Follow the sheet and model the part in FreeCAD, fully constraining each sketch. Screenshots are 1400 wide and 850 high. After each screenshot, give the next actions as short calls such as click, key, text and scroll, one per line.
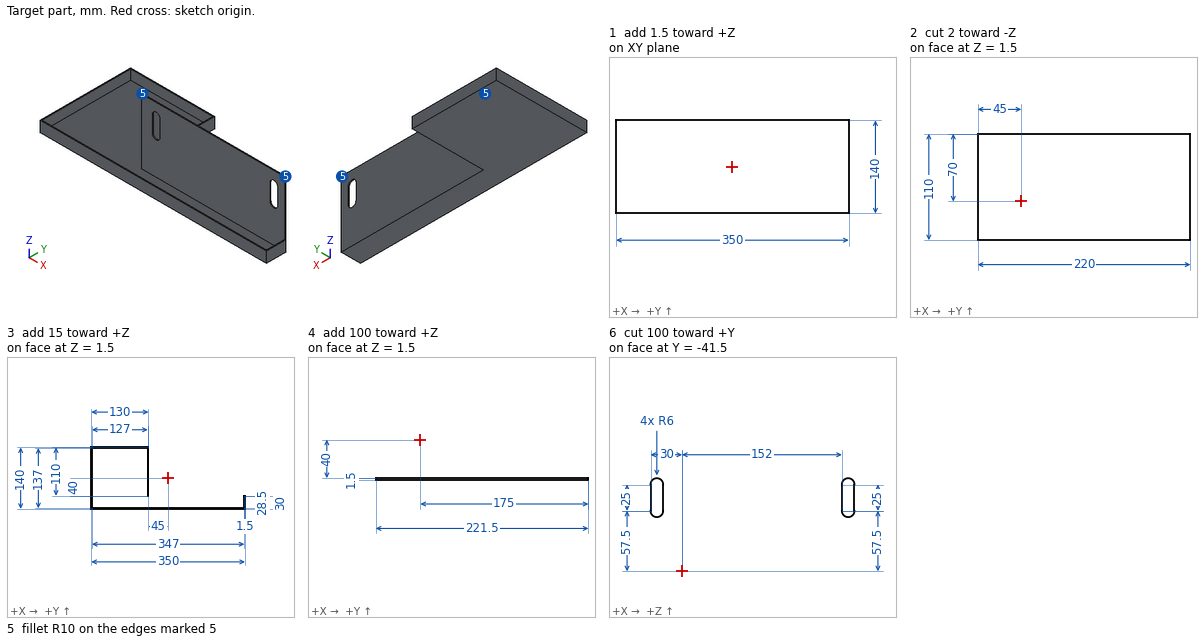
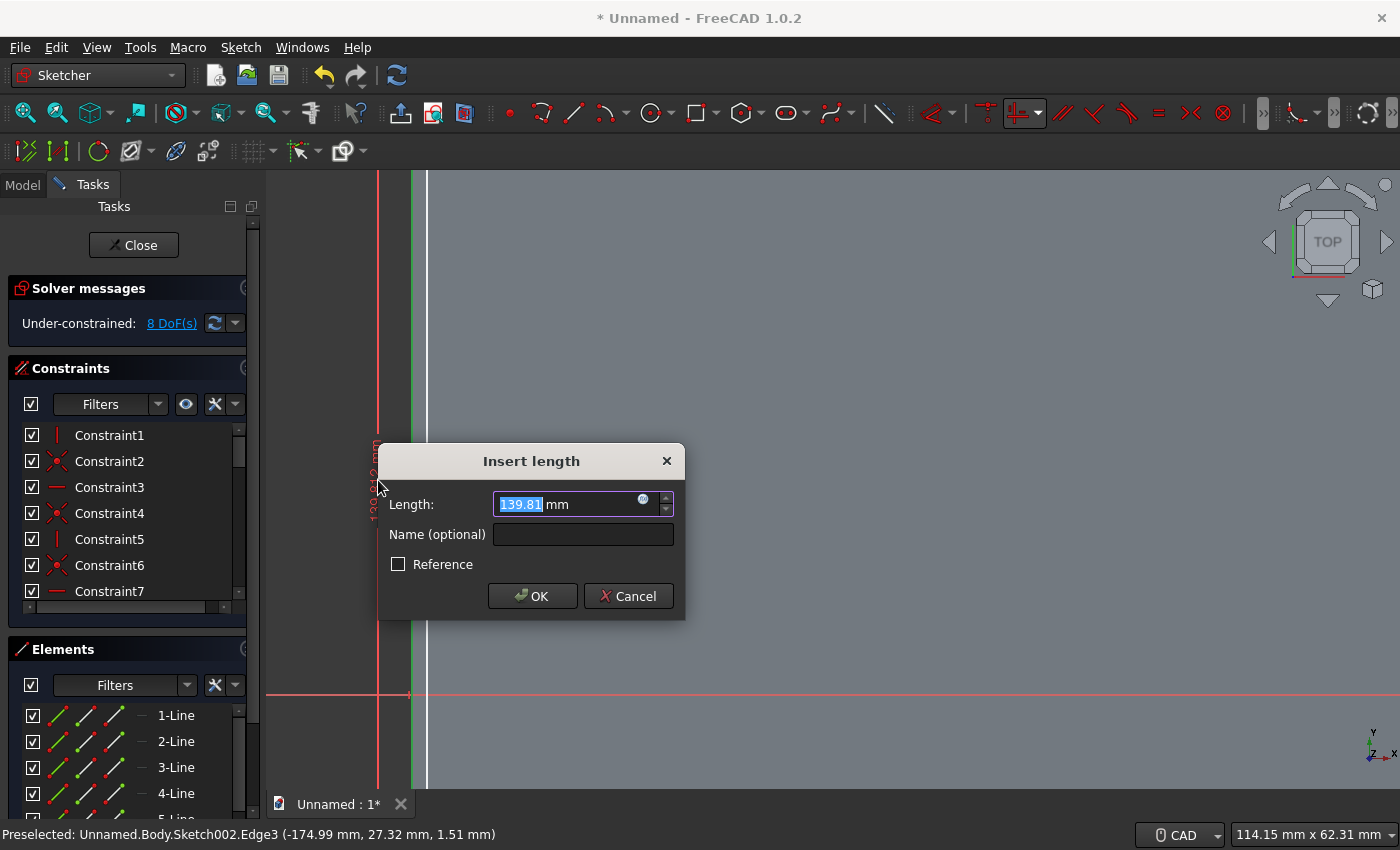
text(140)
key(Return)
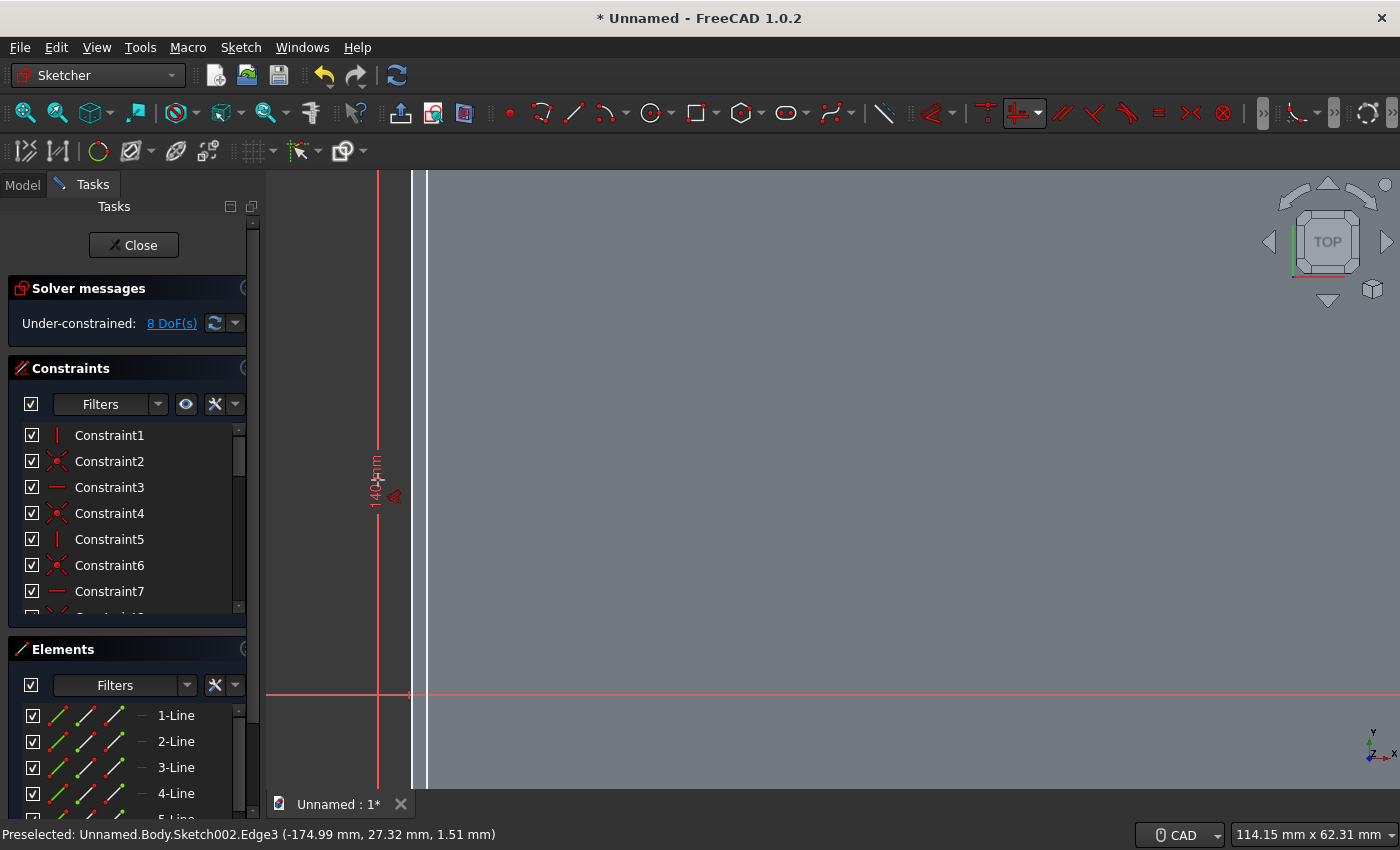
scroll(414, 425, down, 8)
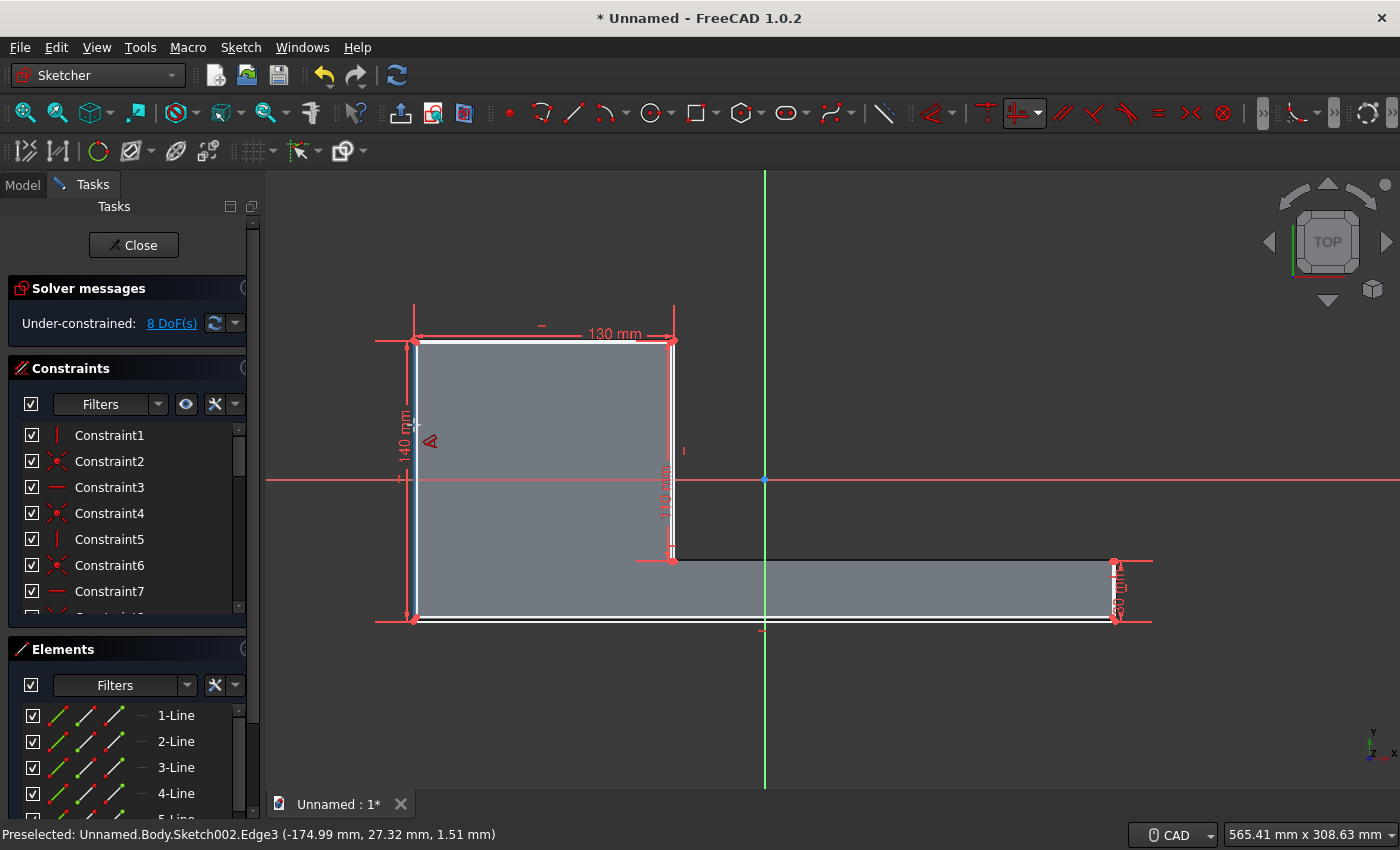
scroll(624, 622, up, 7)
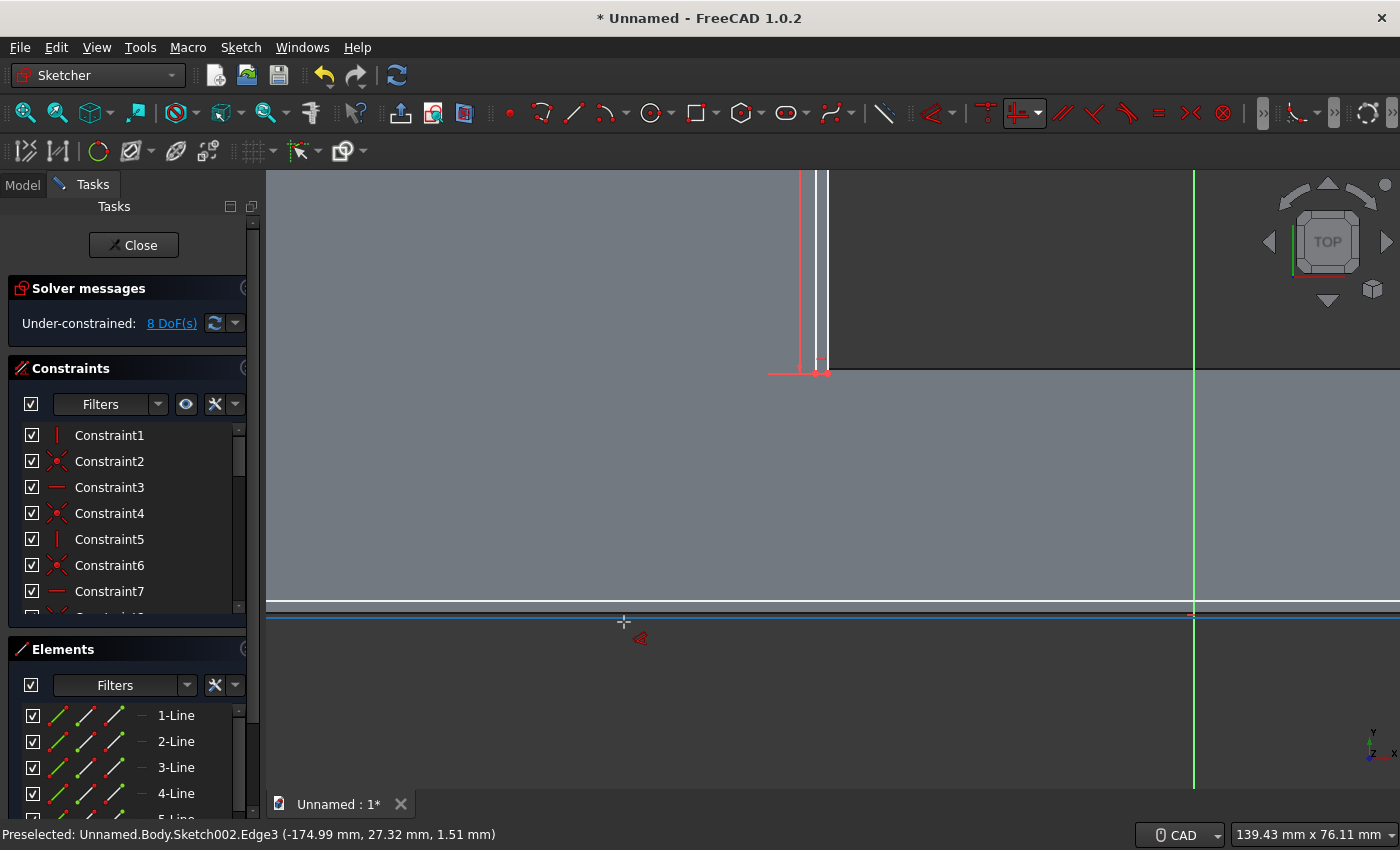
click(624, 618)
click(764, 652)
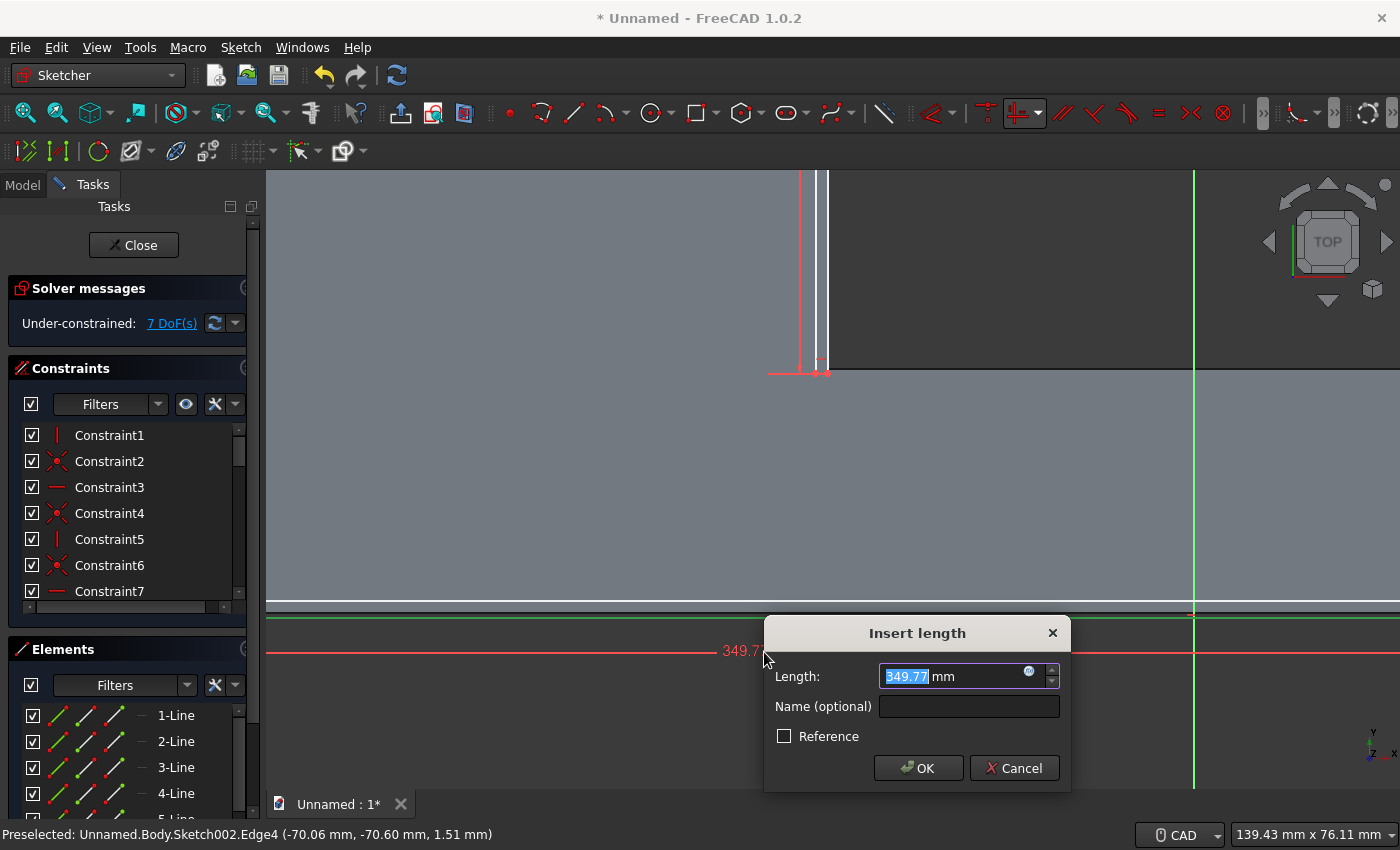
text(350)
key(Return)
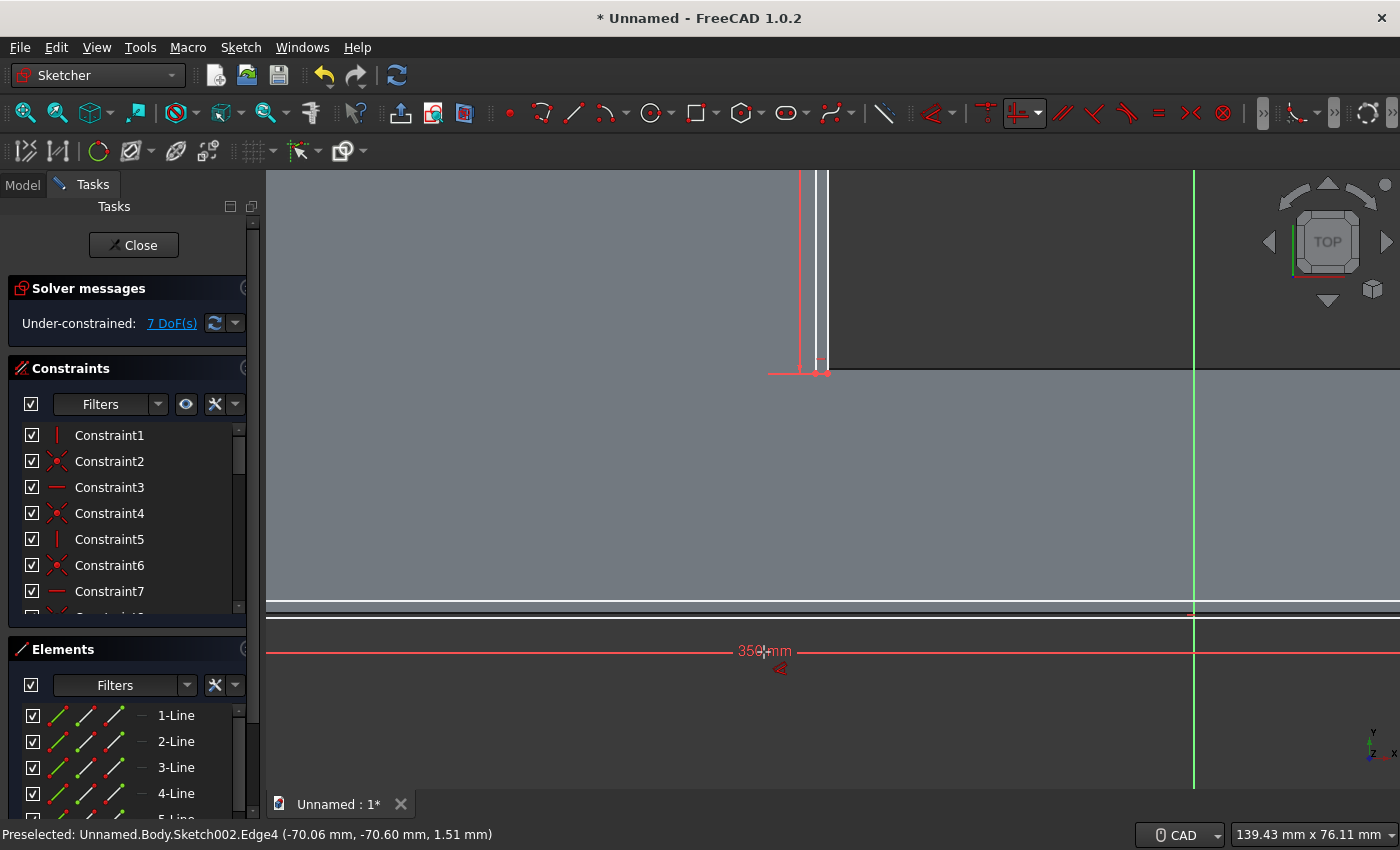
scroll(624, 622, down, 7)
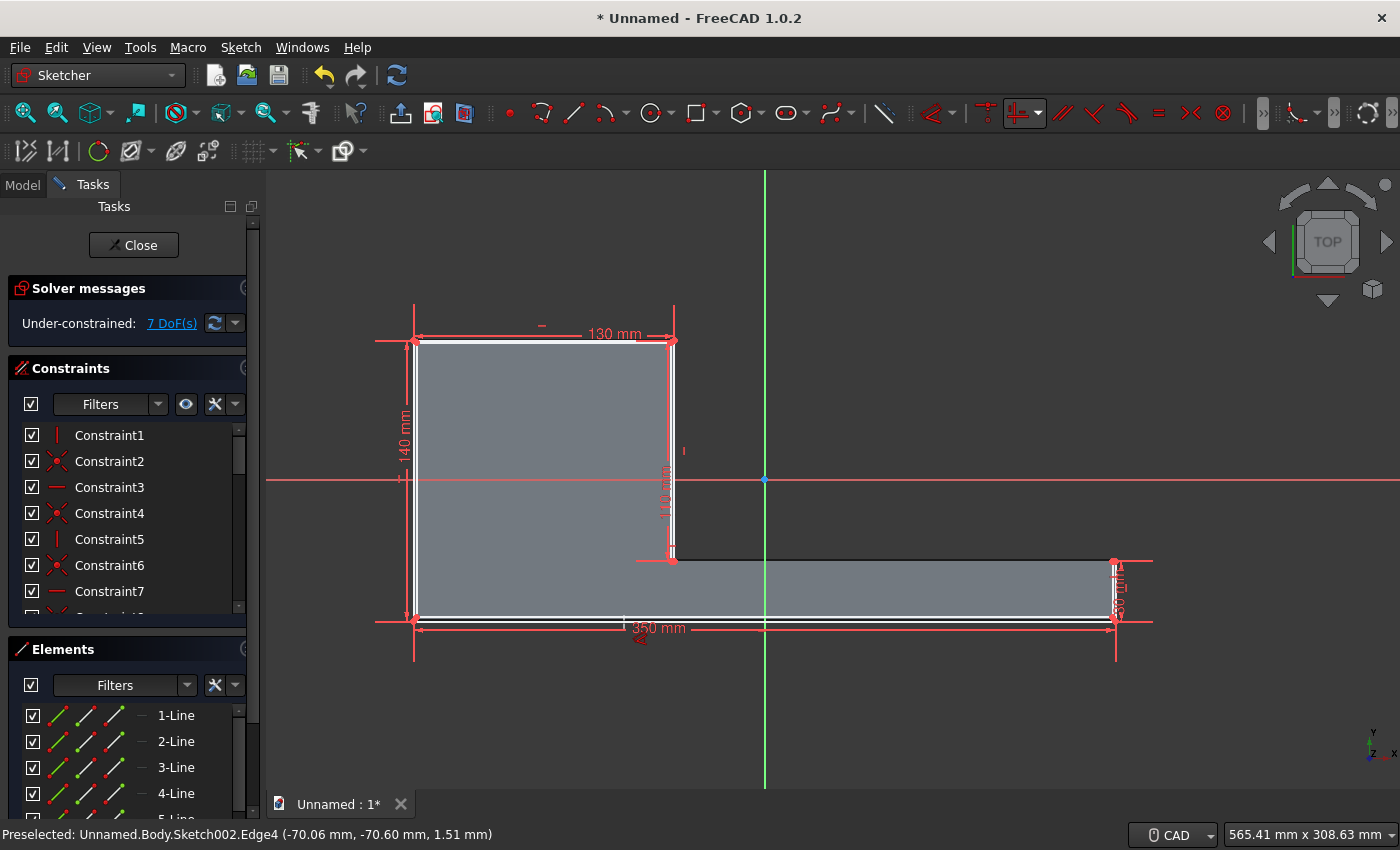
scroll(1114, 561, up, 13)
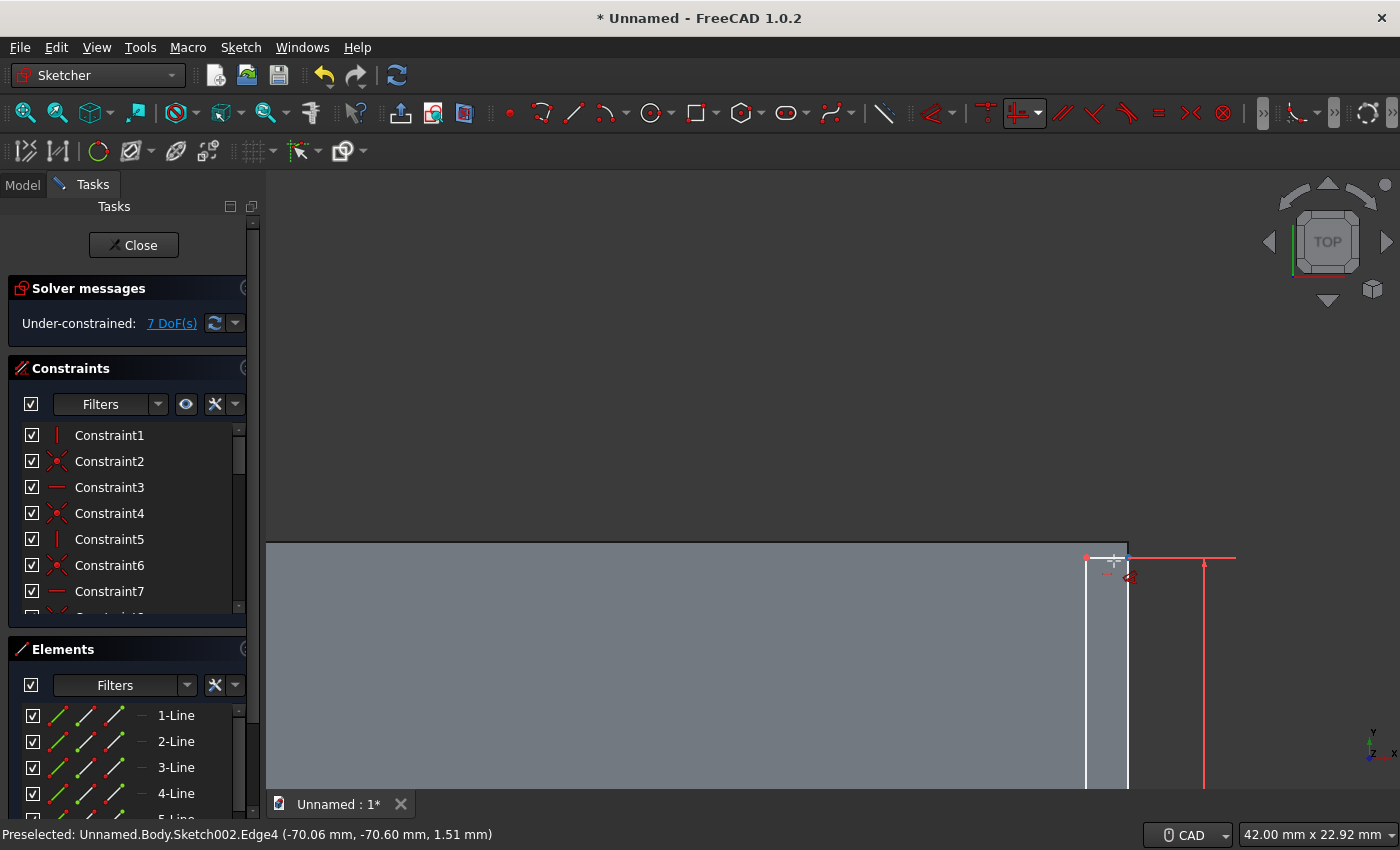
click(1107, 558)
click(1107, 592)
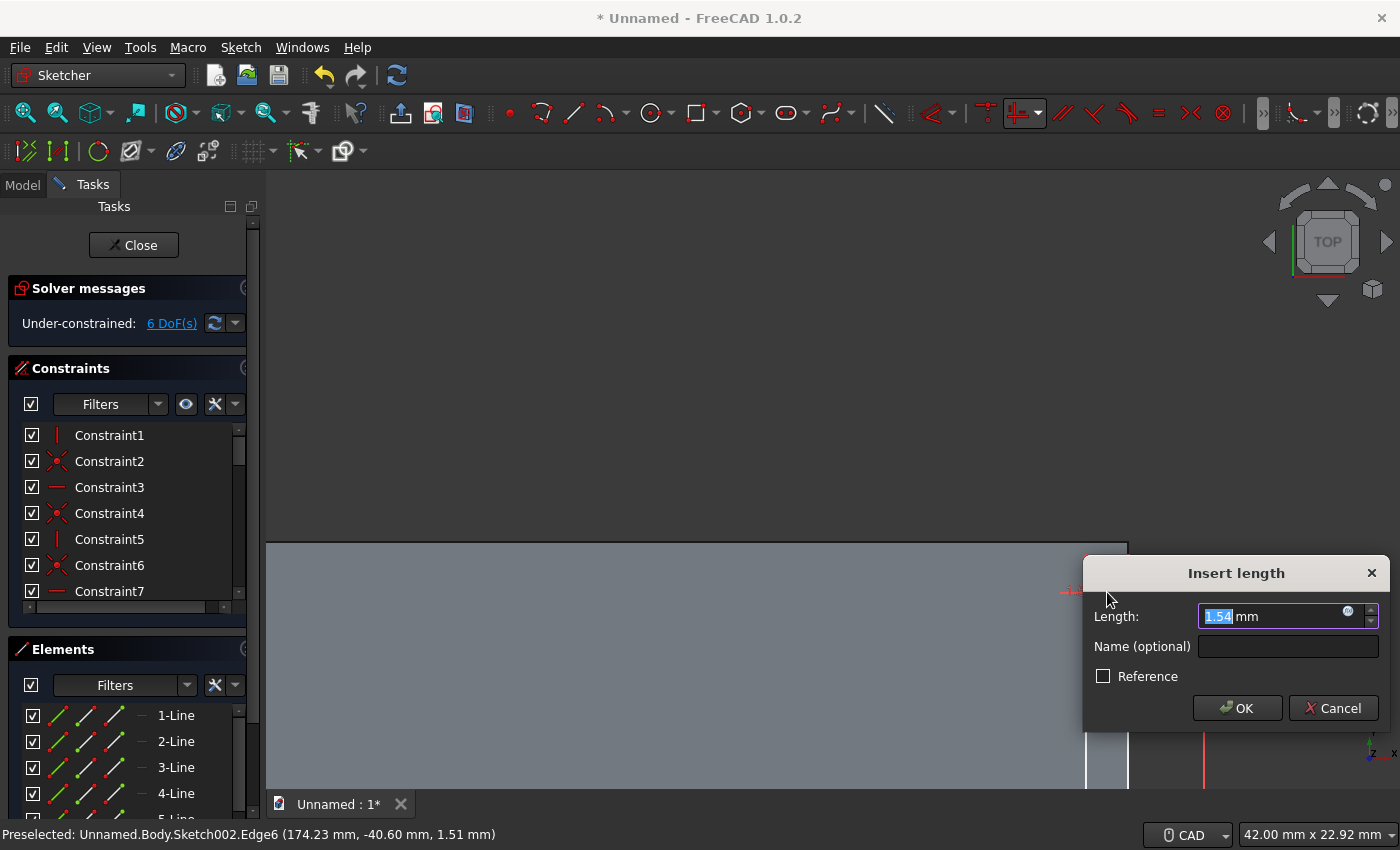
text(1.5)
key(Return)